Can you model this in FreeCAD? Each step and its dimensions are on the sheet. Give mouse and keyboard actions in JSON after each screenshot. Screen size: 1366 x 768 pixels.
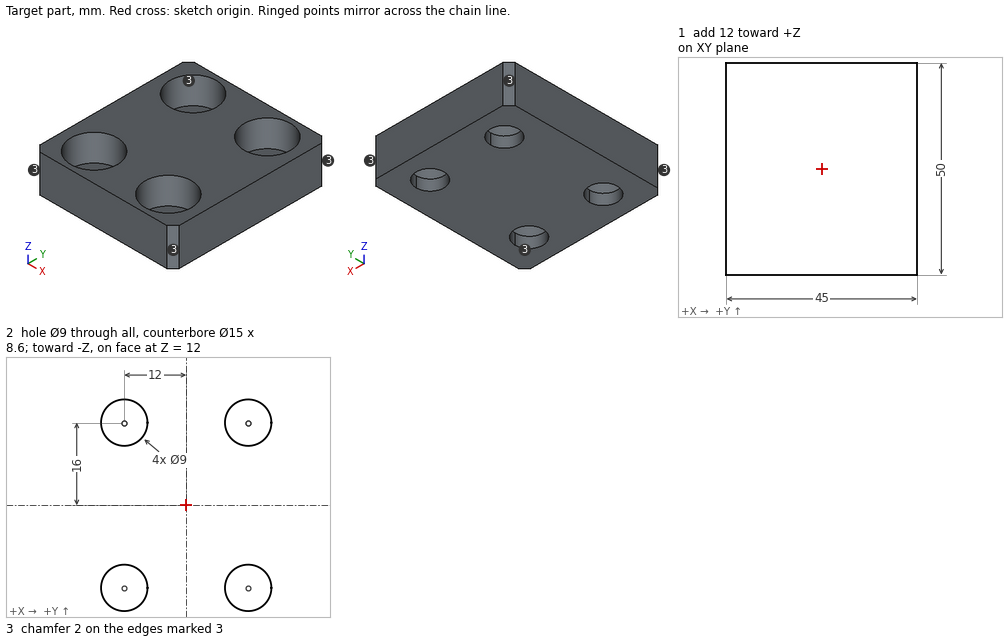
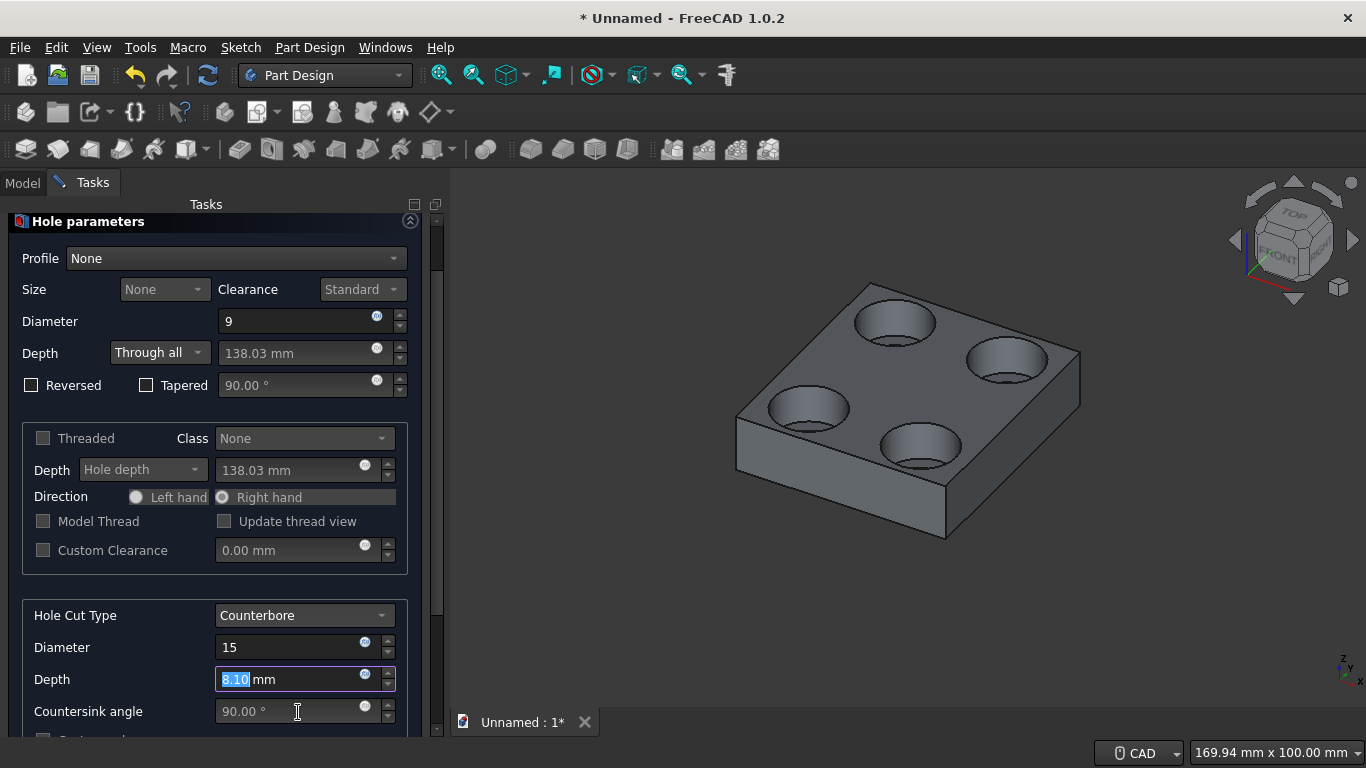
{"action": "type", "text": "8.6"}
{"action": "key", "text": "Tab"}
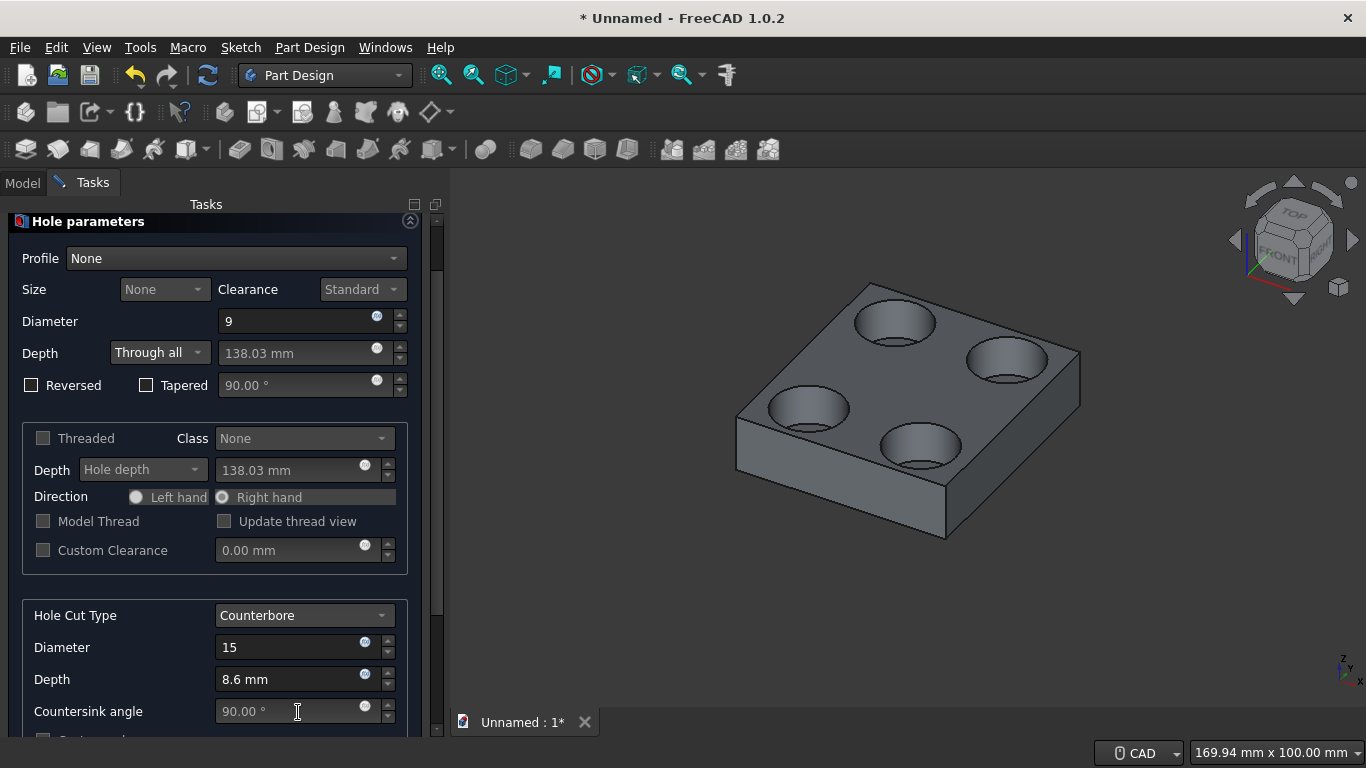
{"action": "scroll", "coordinate": [437, 475], "scroll_direction": "up", "scroll_amount": 2}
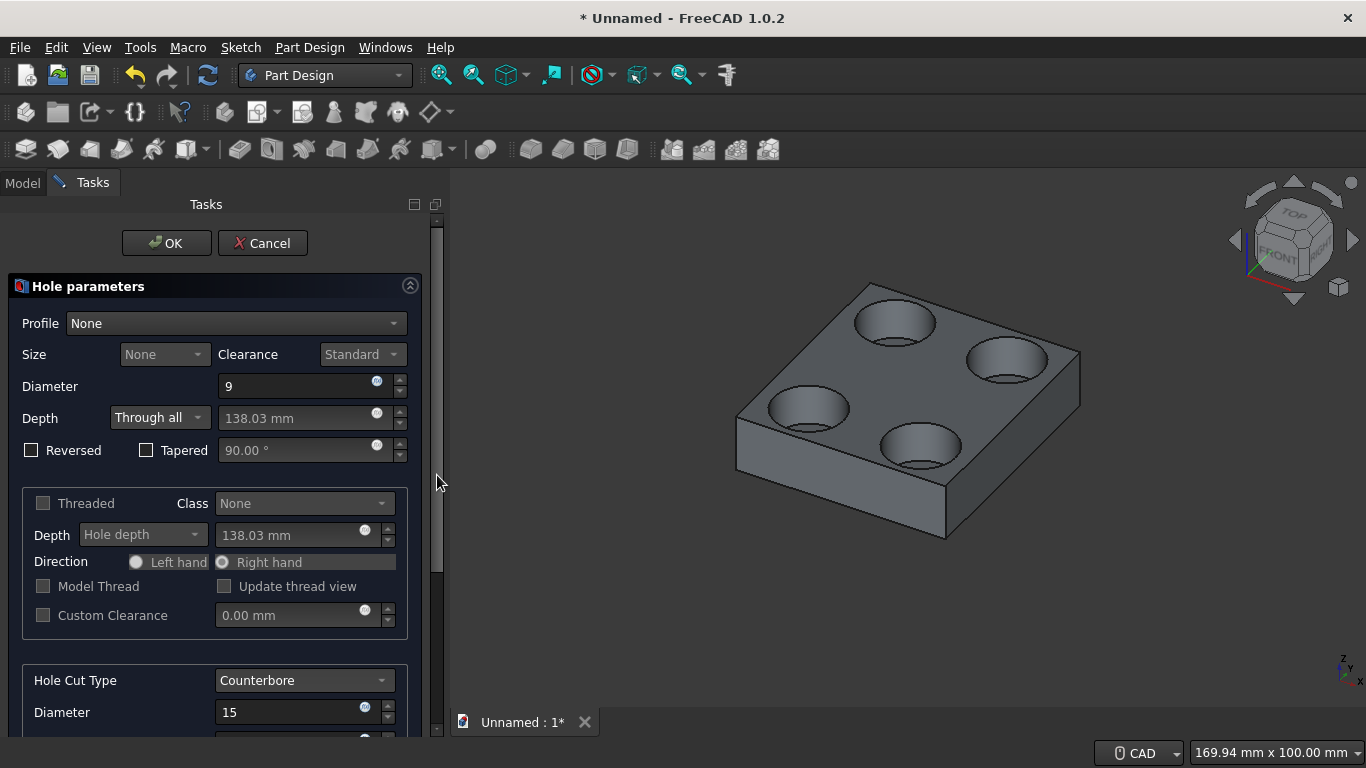
{"action": "left_click", "coordinate": [167, 243]}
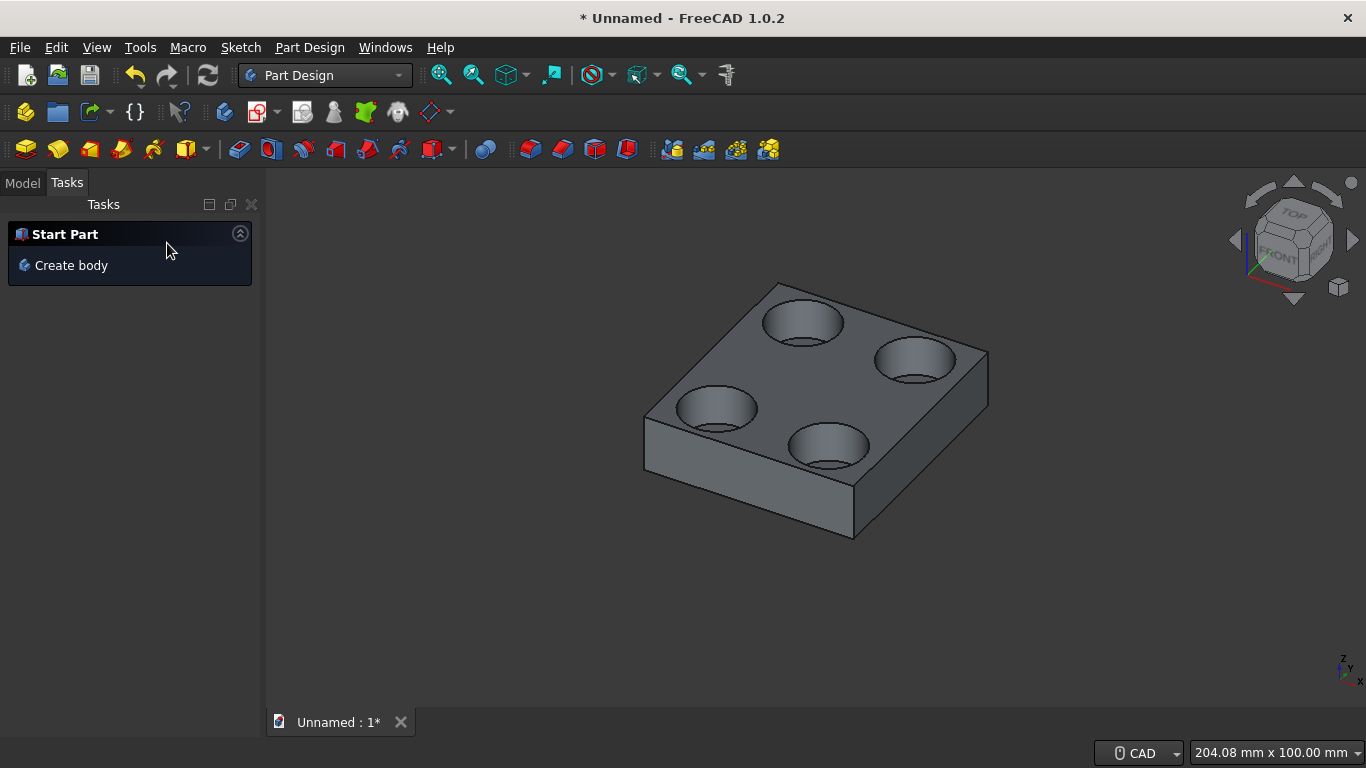
{"action": "left_click", "coordinate": [854, 512]}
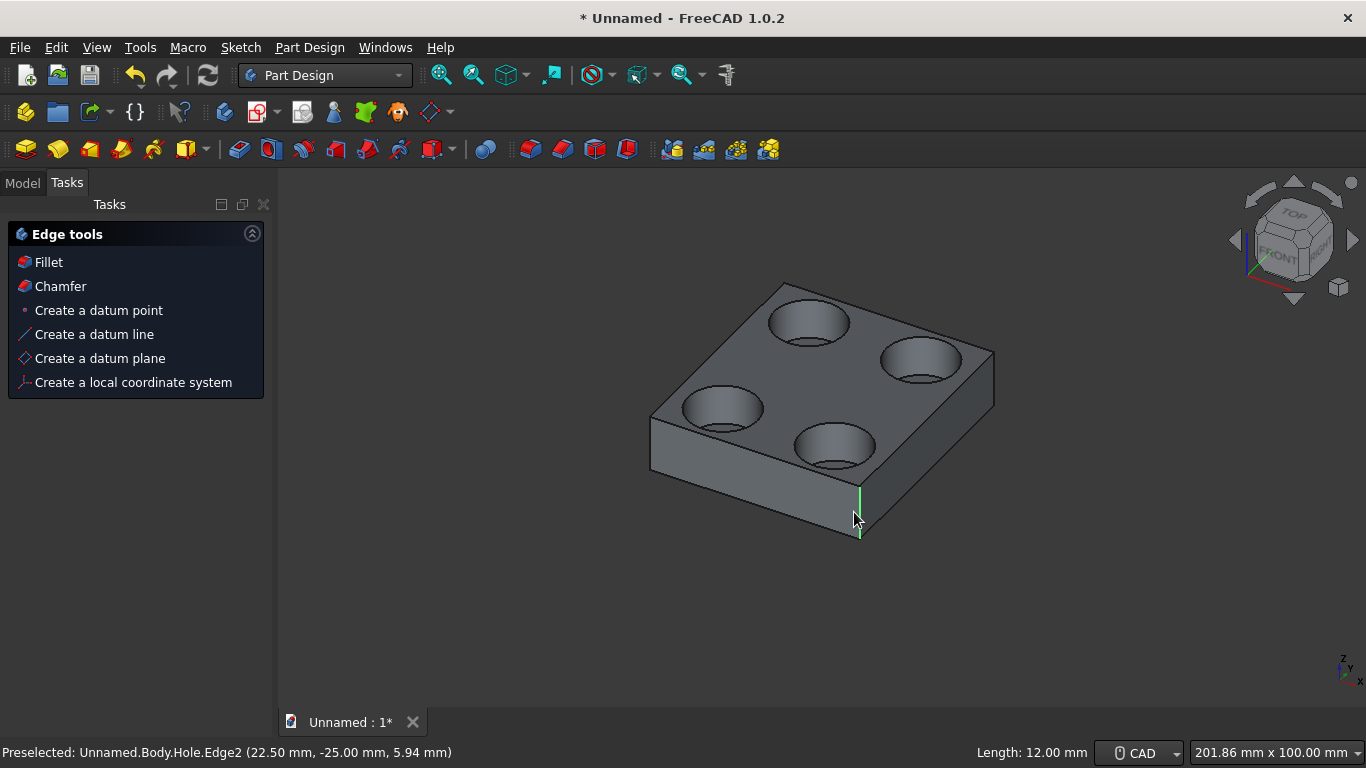
{"action": "key", "text": "0"}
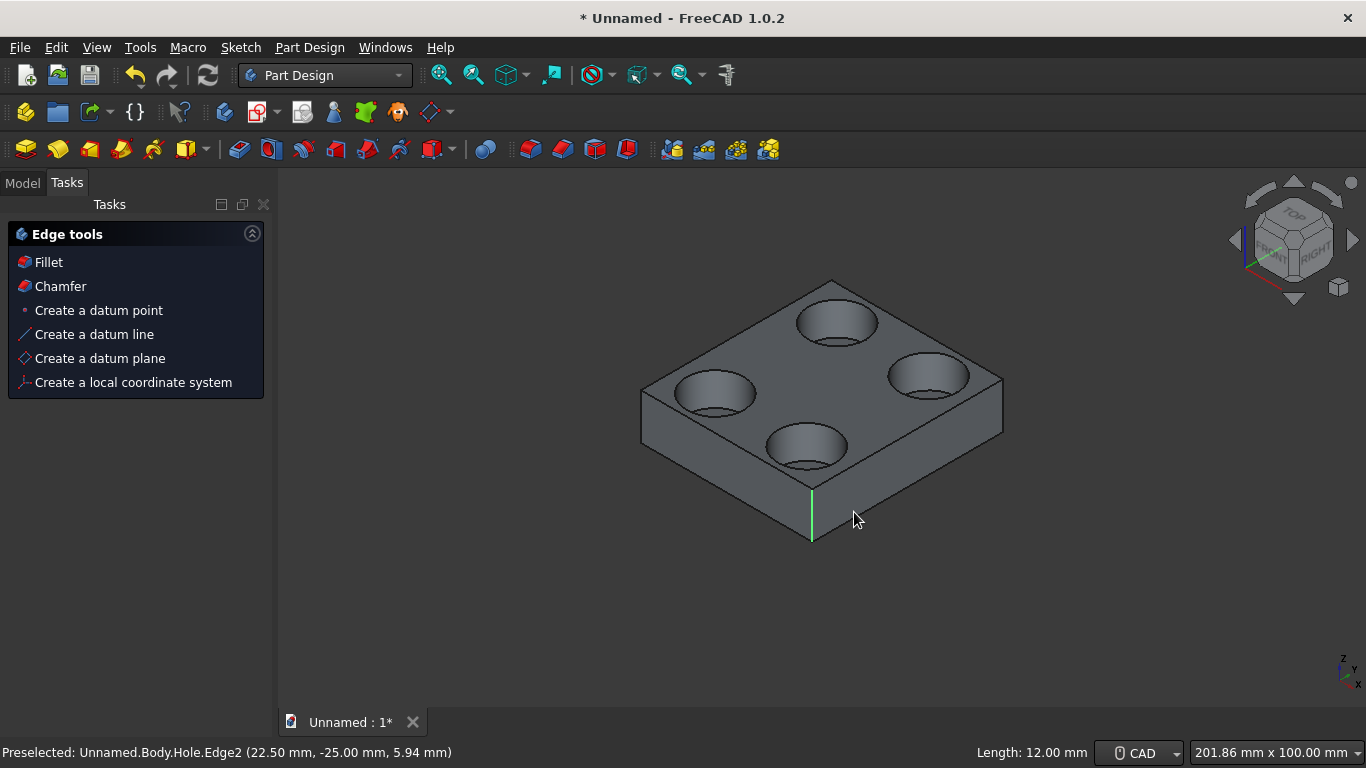
{"action": "key", "text": "2"}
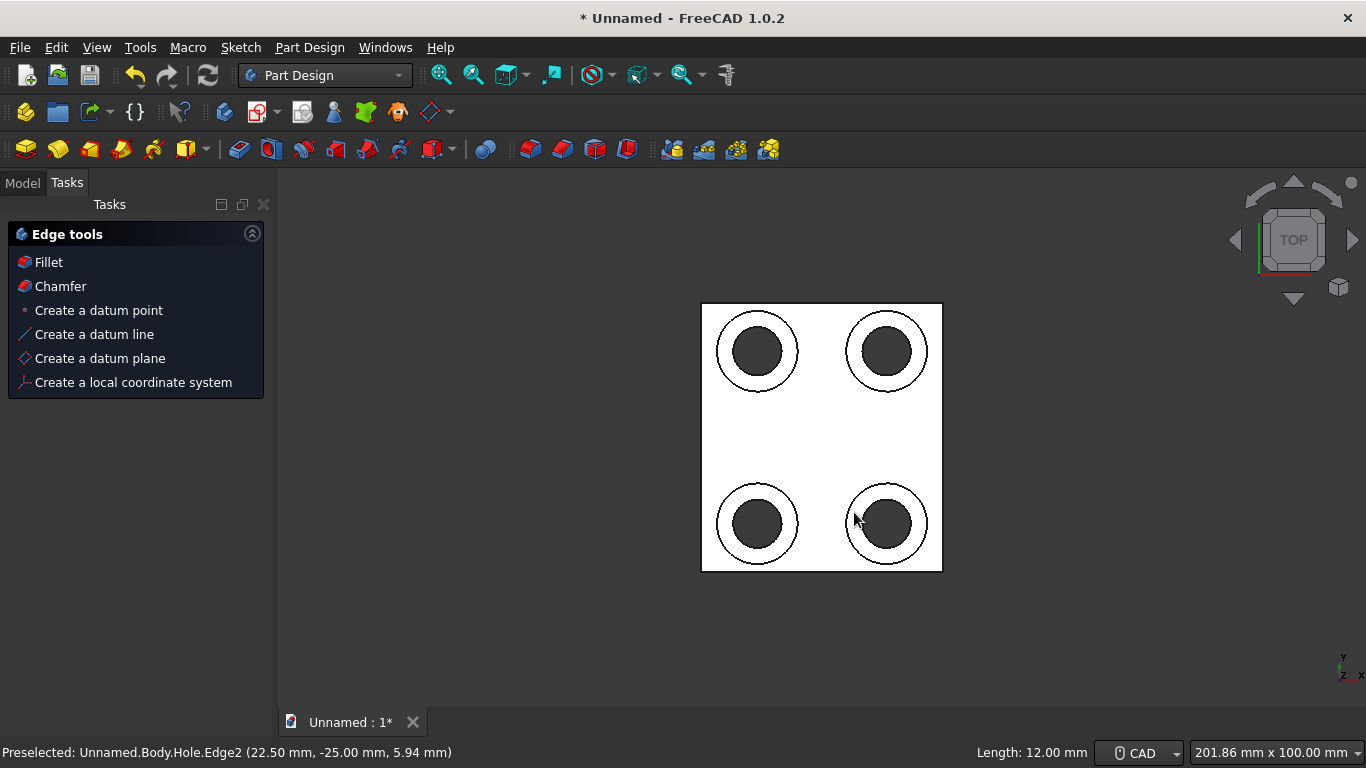
{"action": "key", "text": "1"}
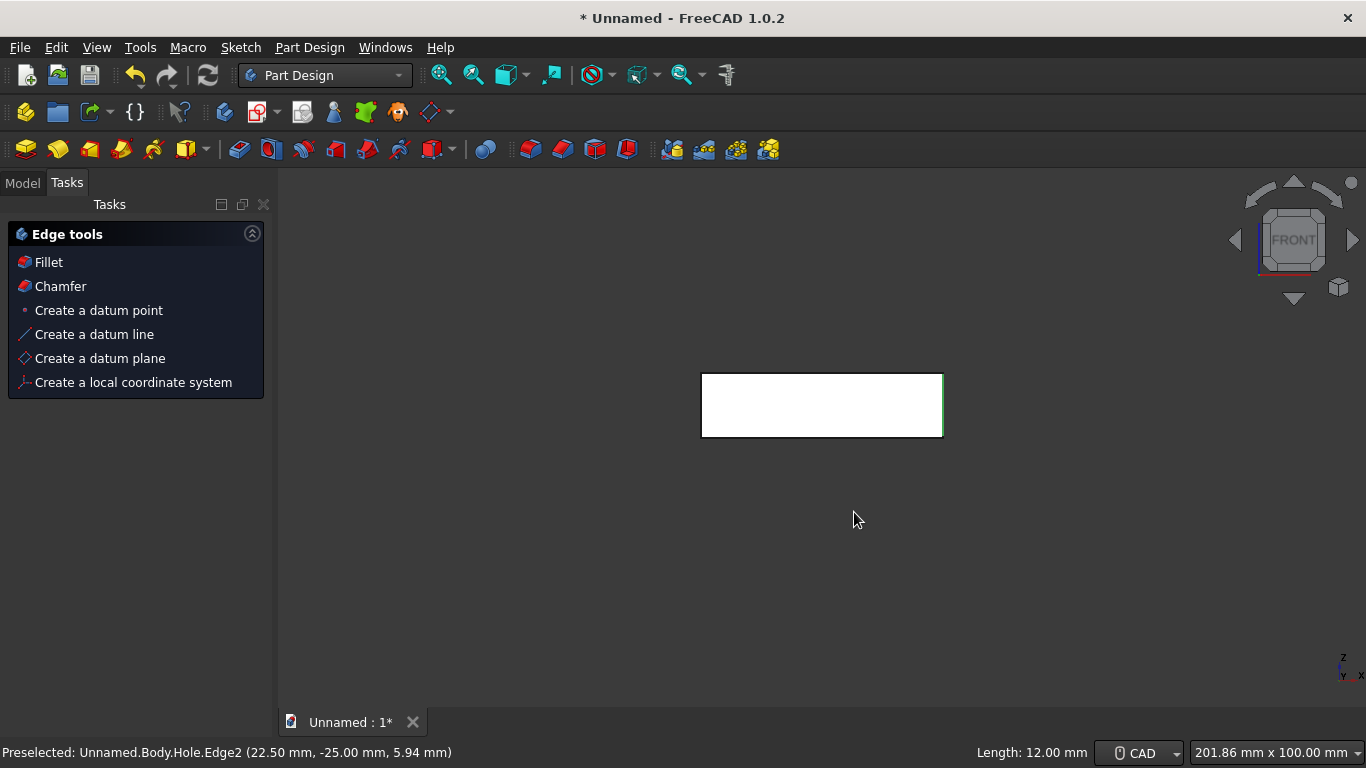
{"action": "left_click", "coordinate": [442, 76]}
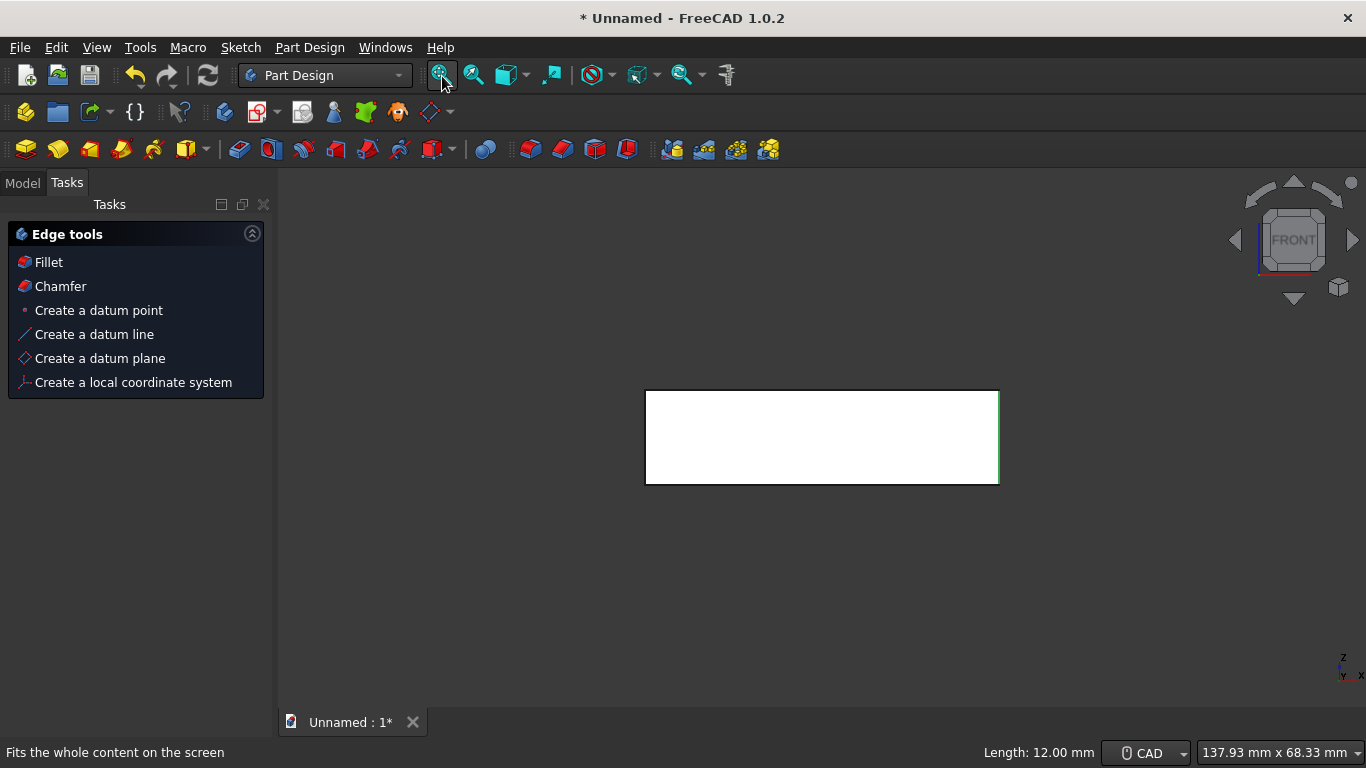
{"action": "left_click", "coordinate": [645, 437], "text": "ctrl"}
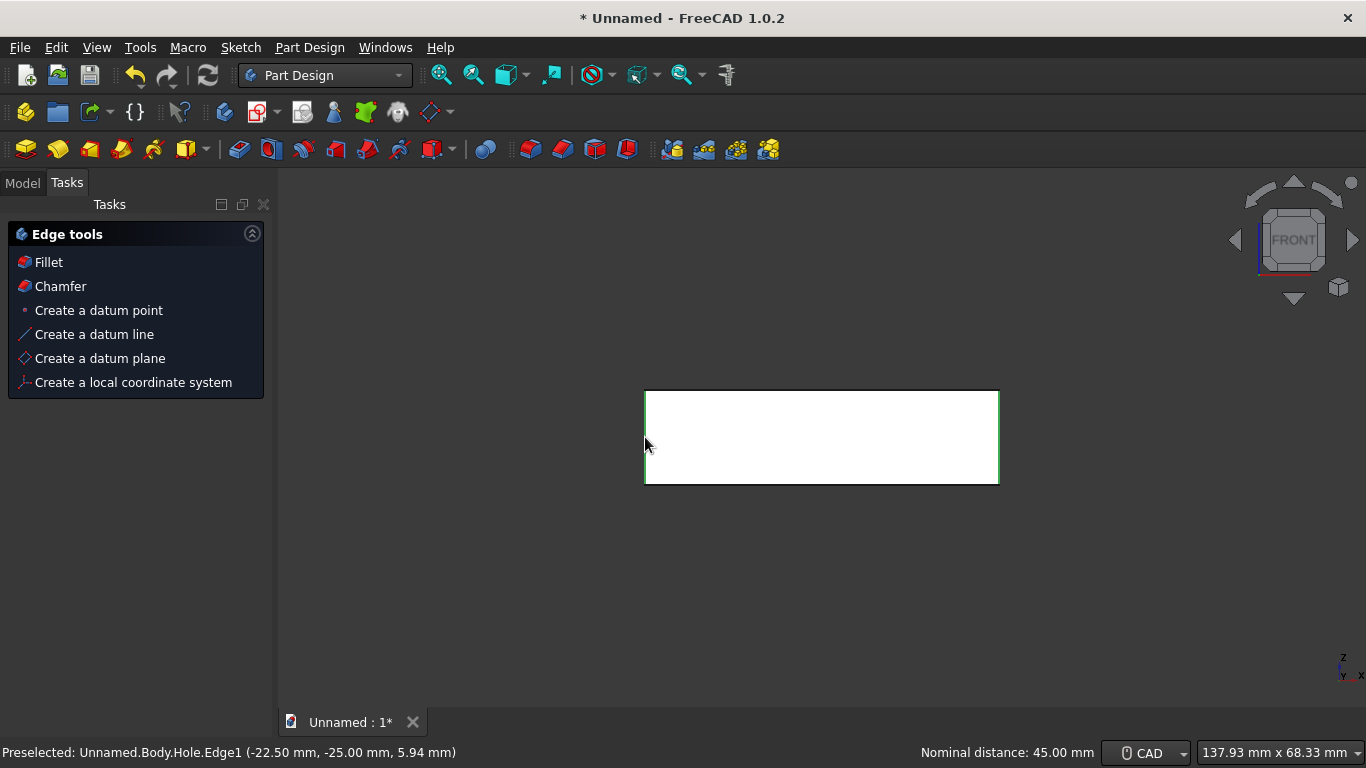
{"action": "key", "text": "3"}